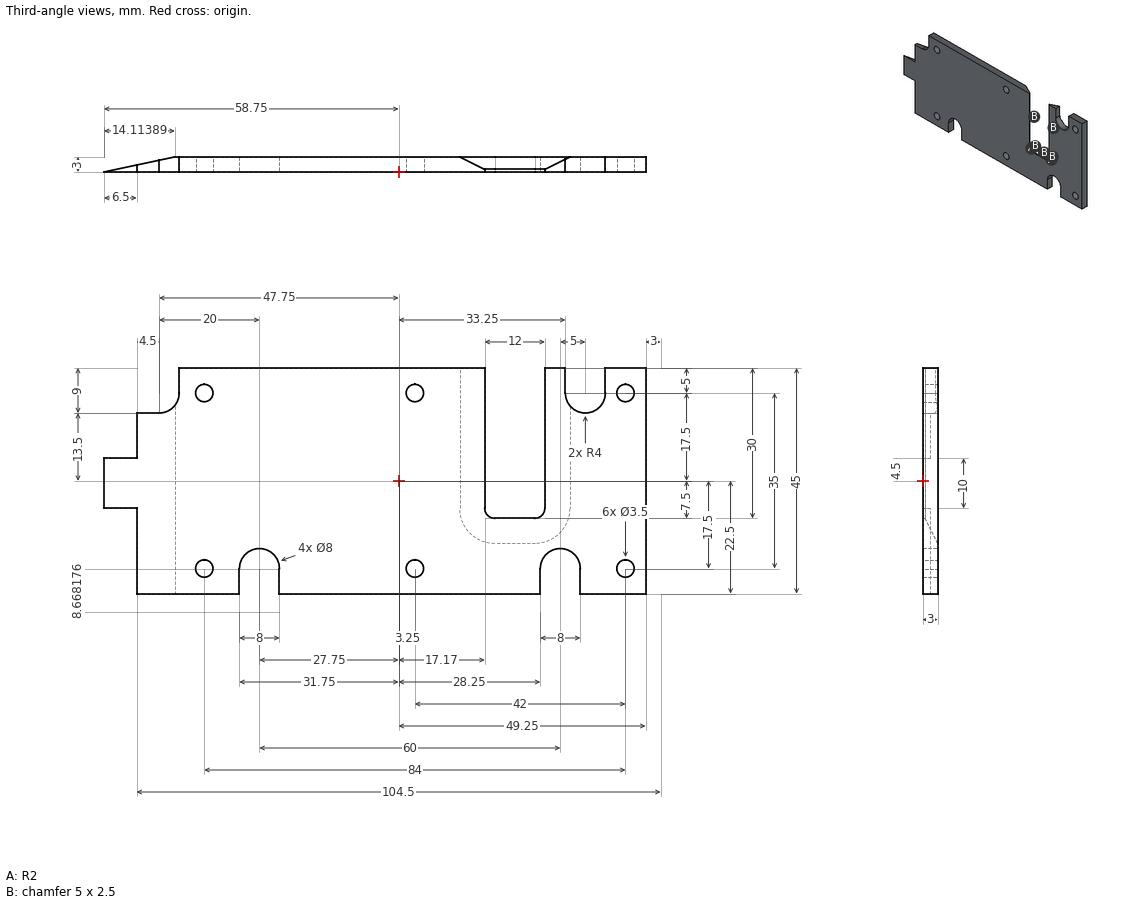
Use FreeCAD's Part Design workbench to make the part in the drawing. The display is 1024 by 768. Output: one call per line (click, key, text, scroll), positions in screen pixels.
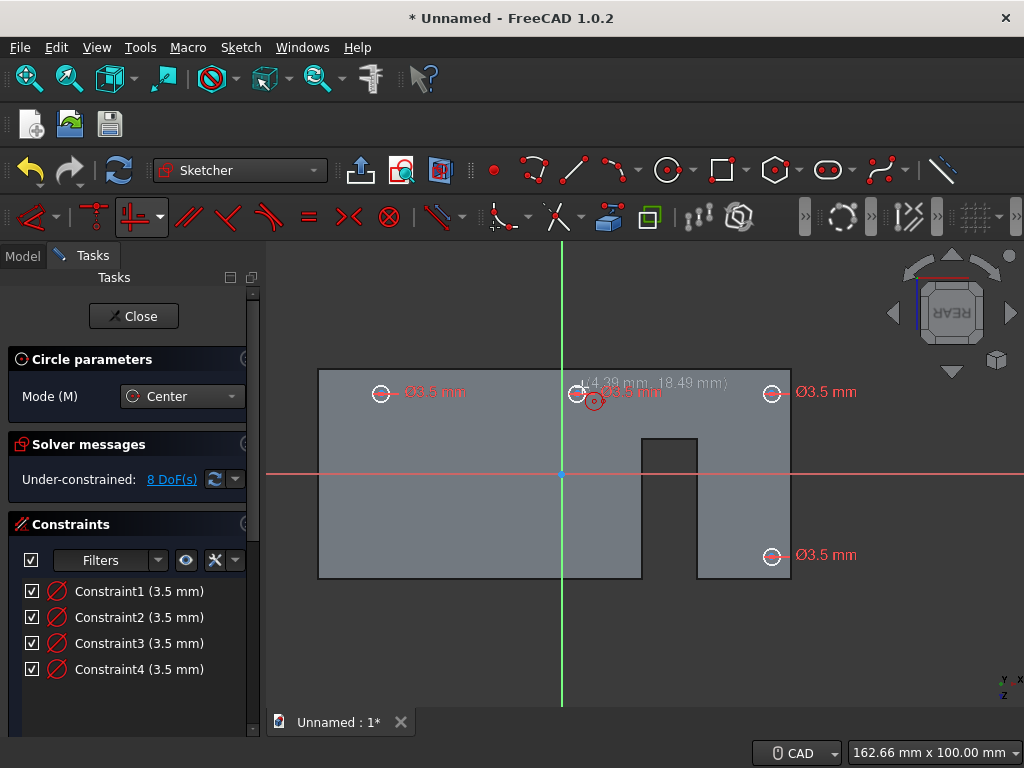
scroll(381, 556, up, 6)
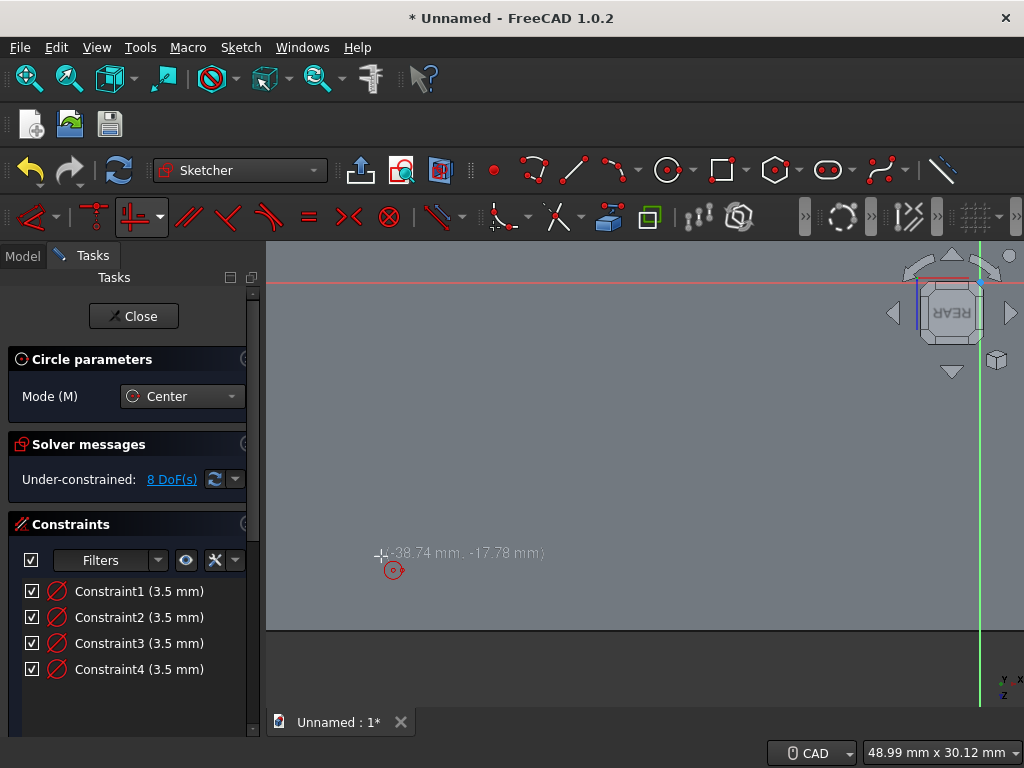
scroll(381, 556, down, 6)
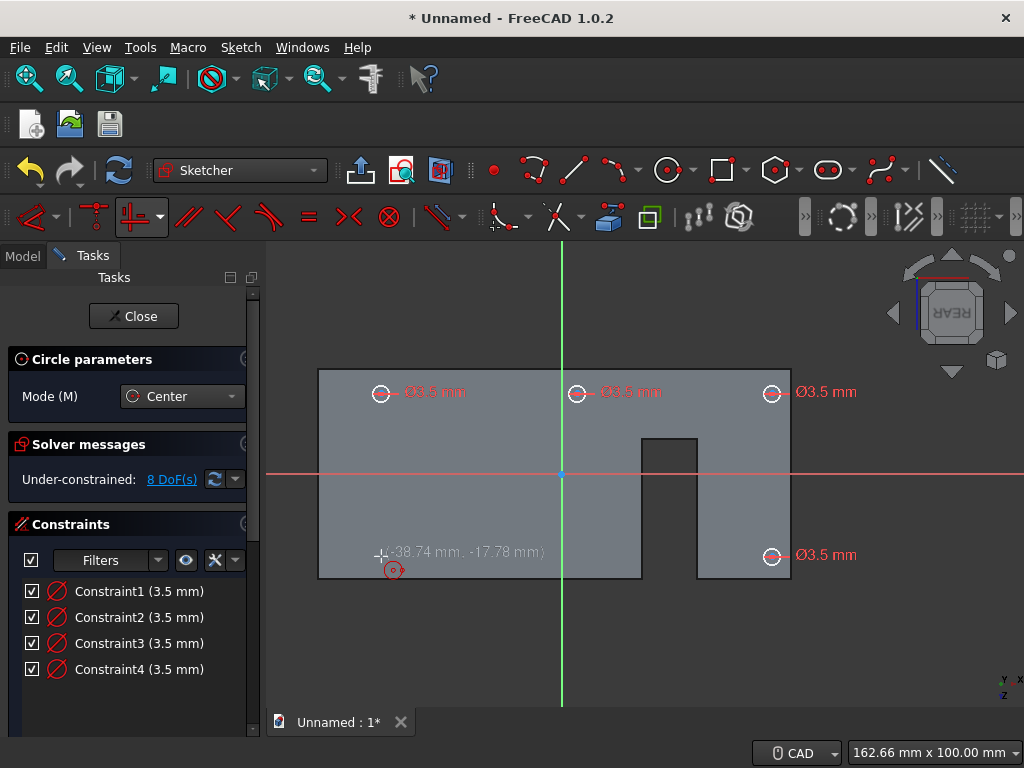
click(381, 556)
move(387, 550)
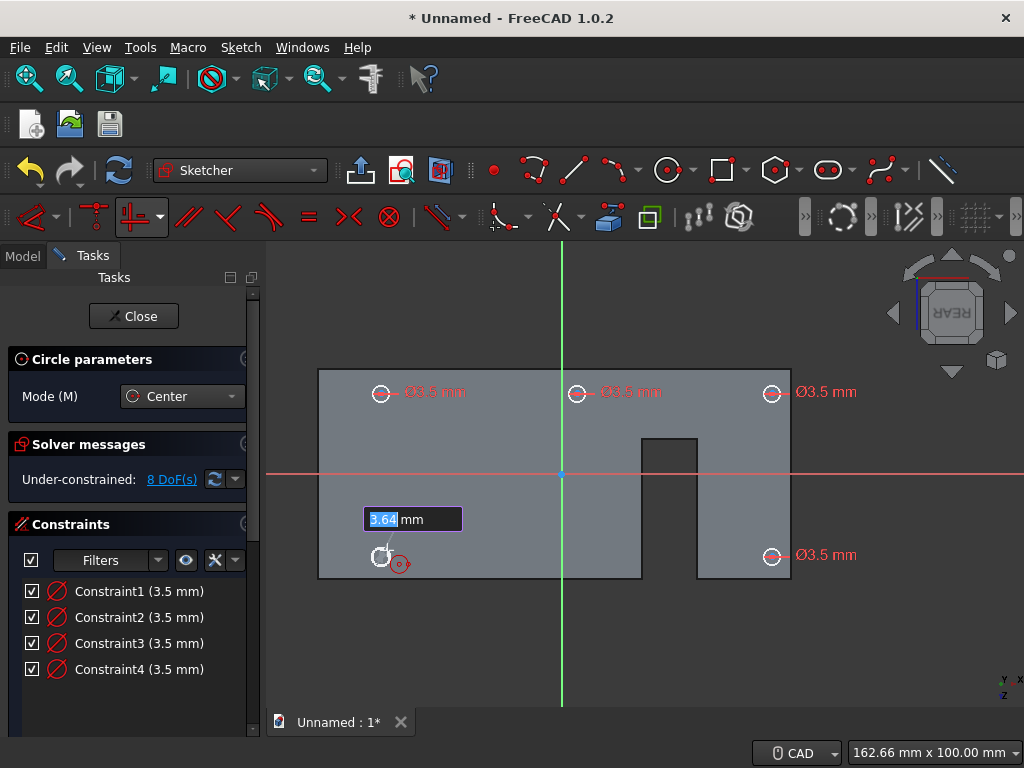
text(3.5)
key(Return)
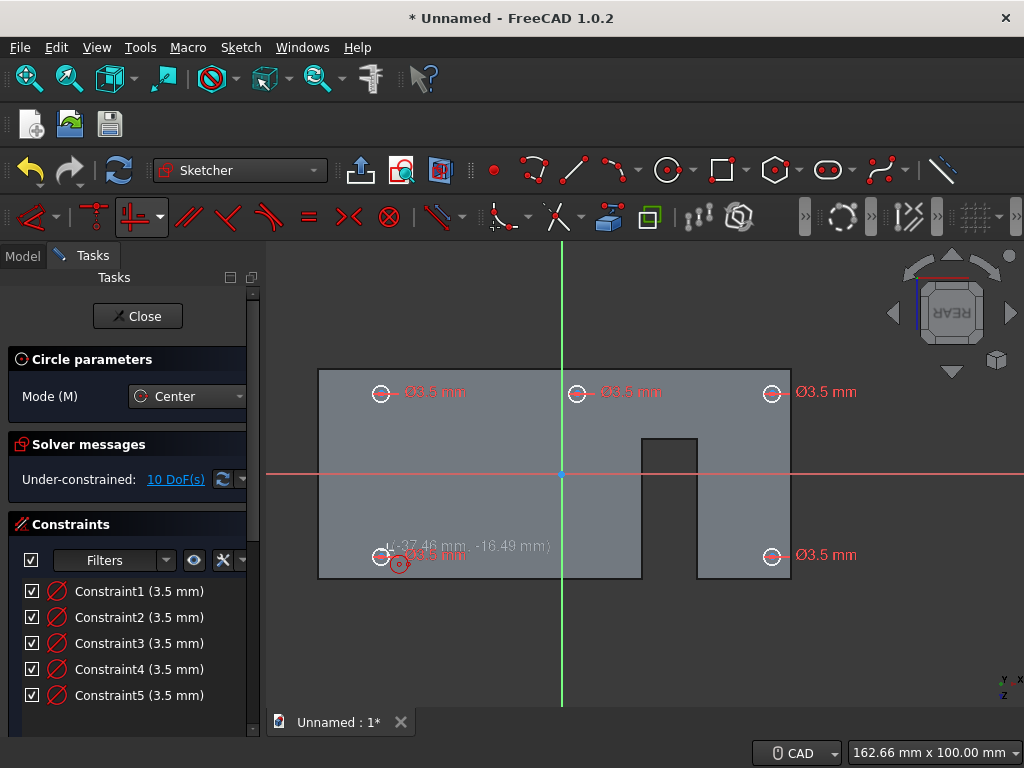
scroll(577, 556, up, 6)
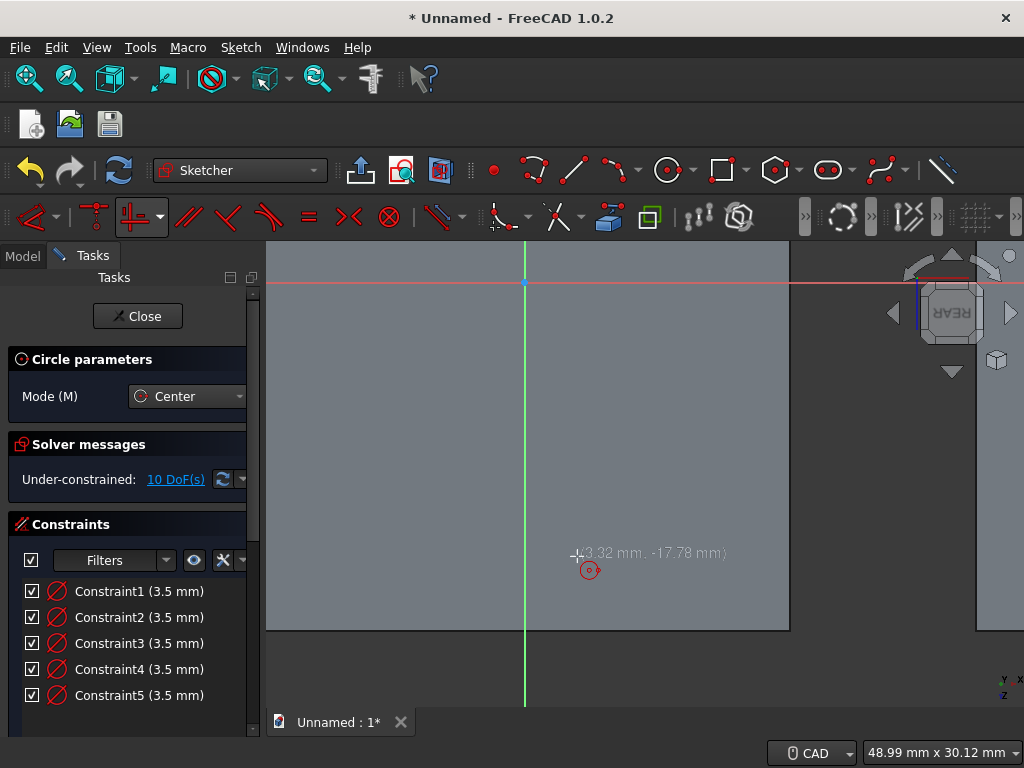
scroll(577, 556, down, 6)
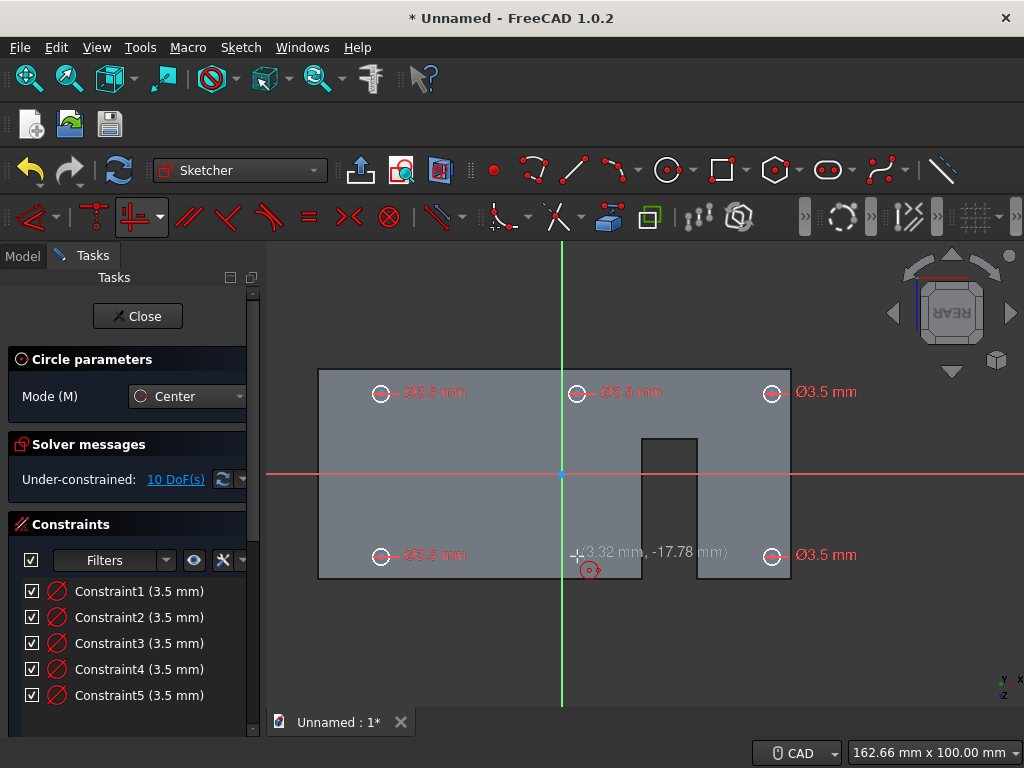
click(577, 556)
move(582, 550)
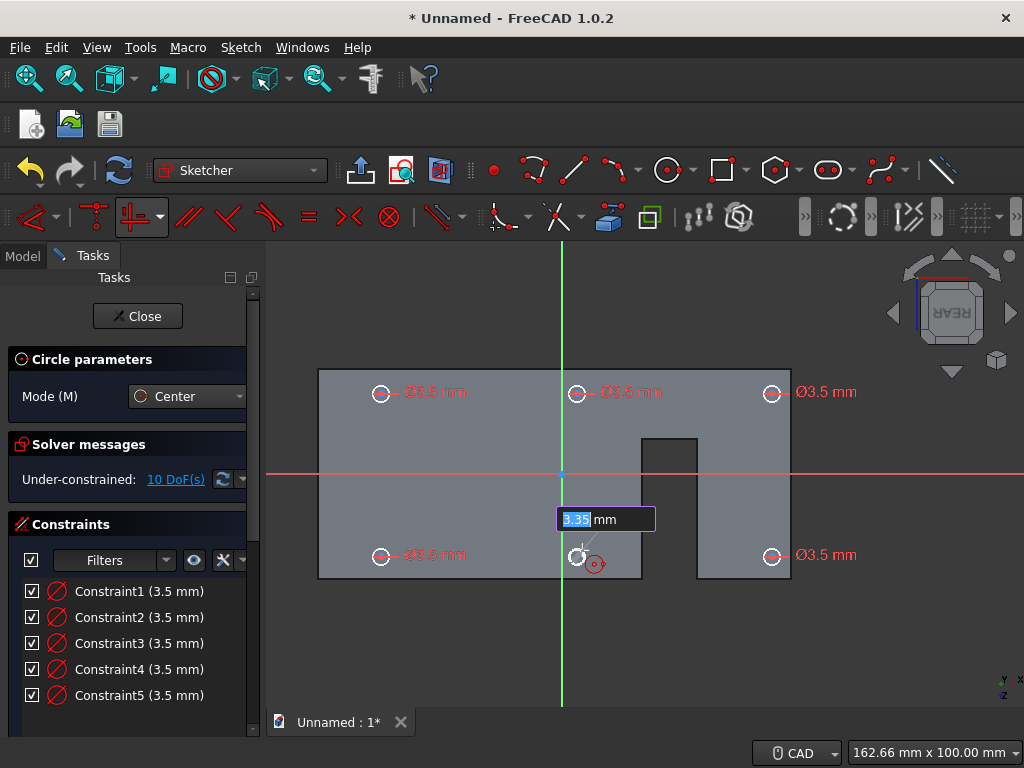
text(3.5)
key(Return)
key(Escape)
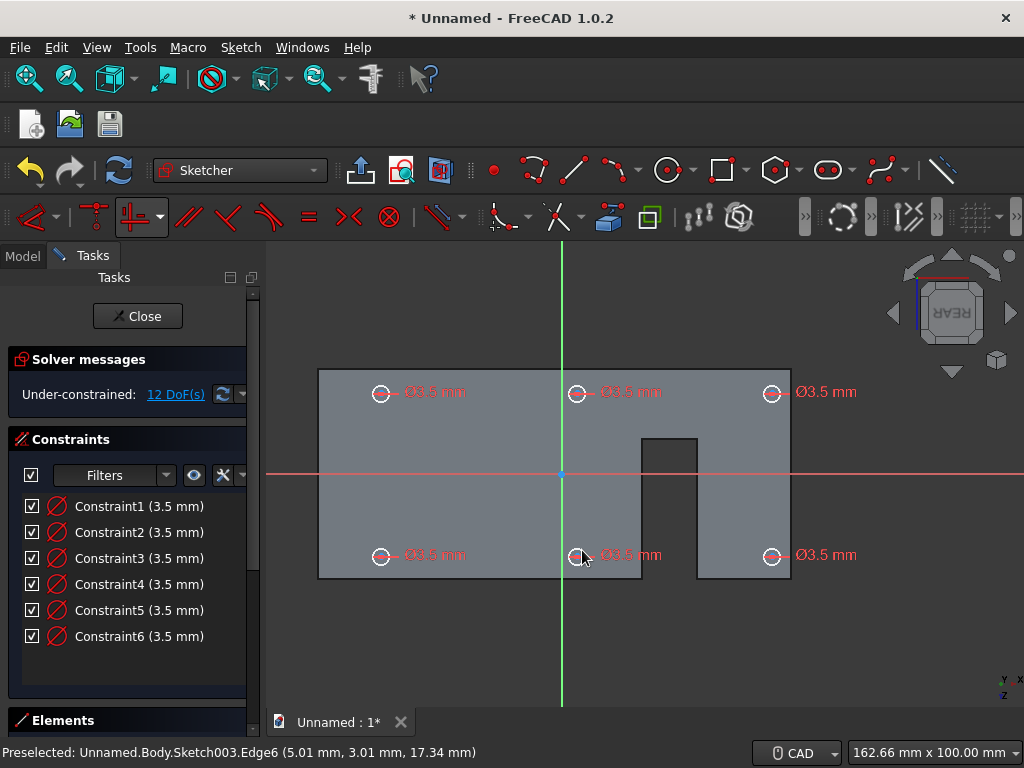
click(772, 394)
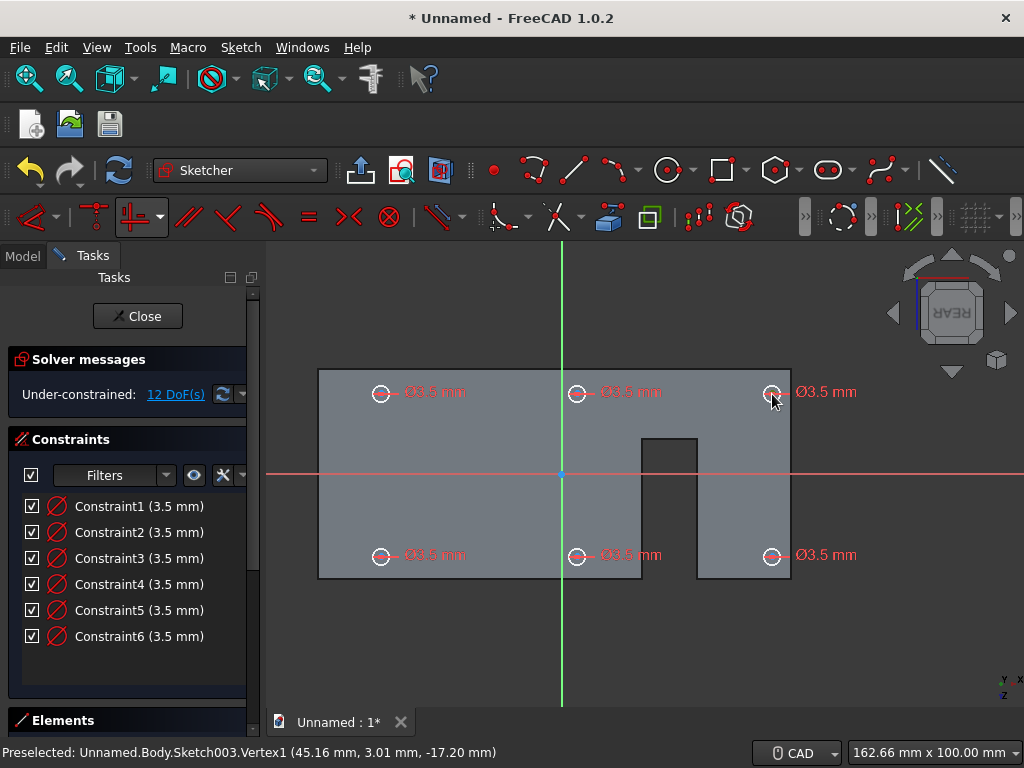
click(772, 557)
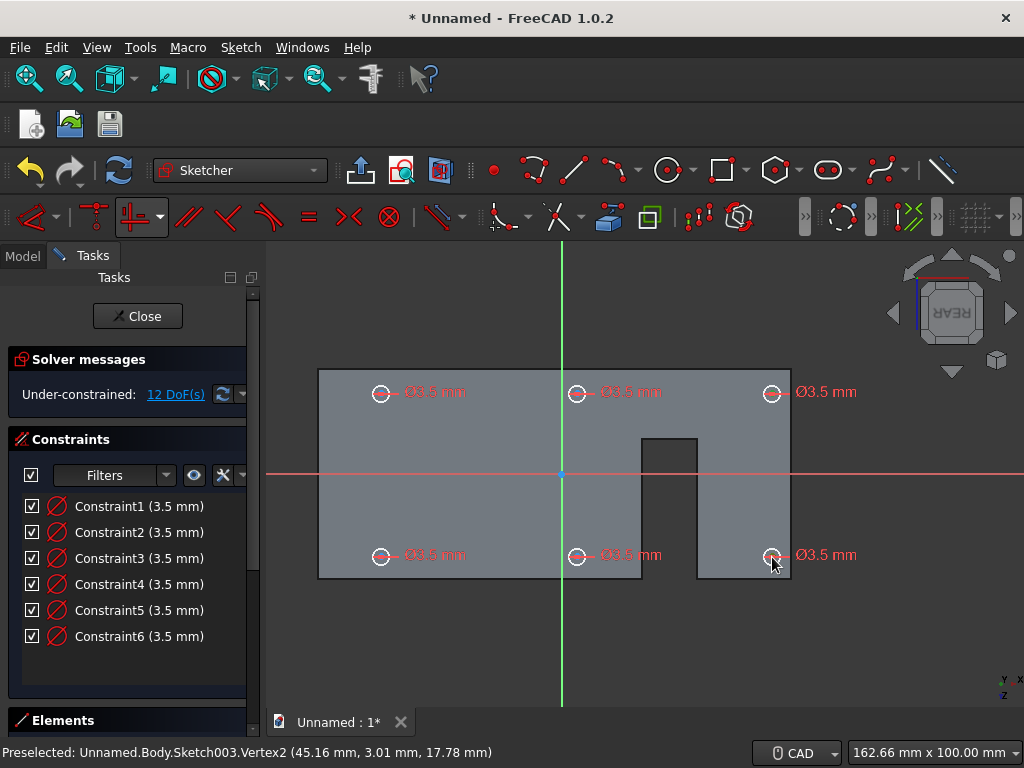
key(v)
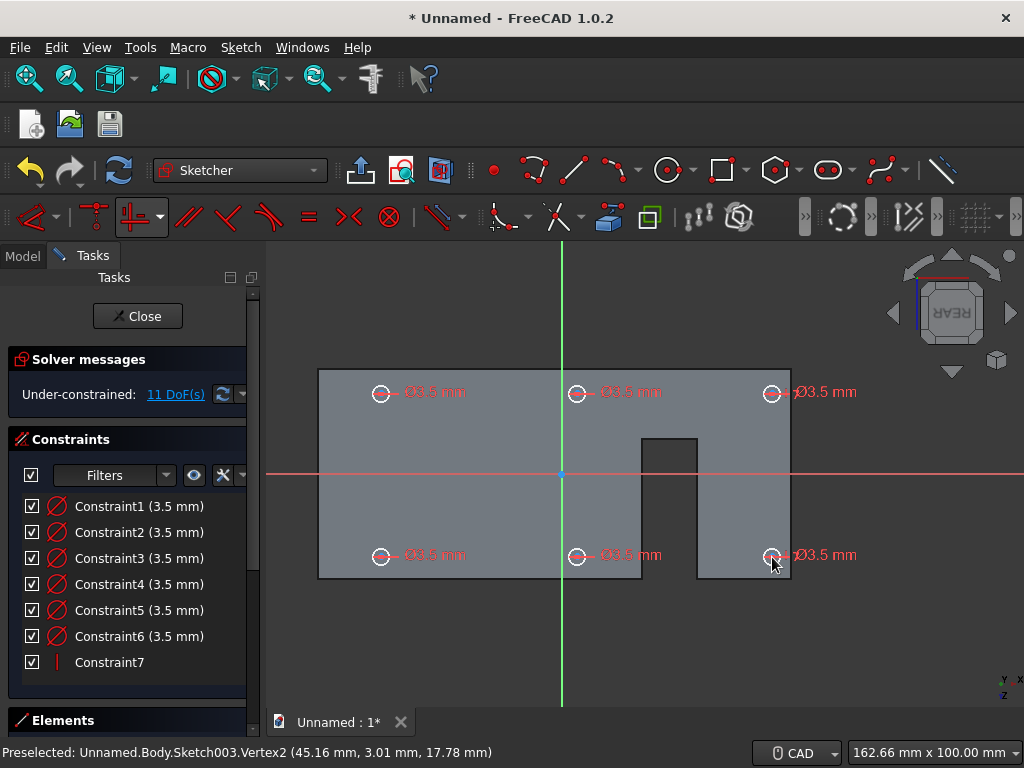
click(772, 394)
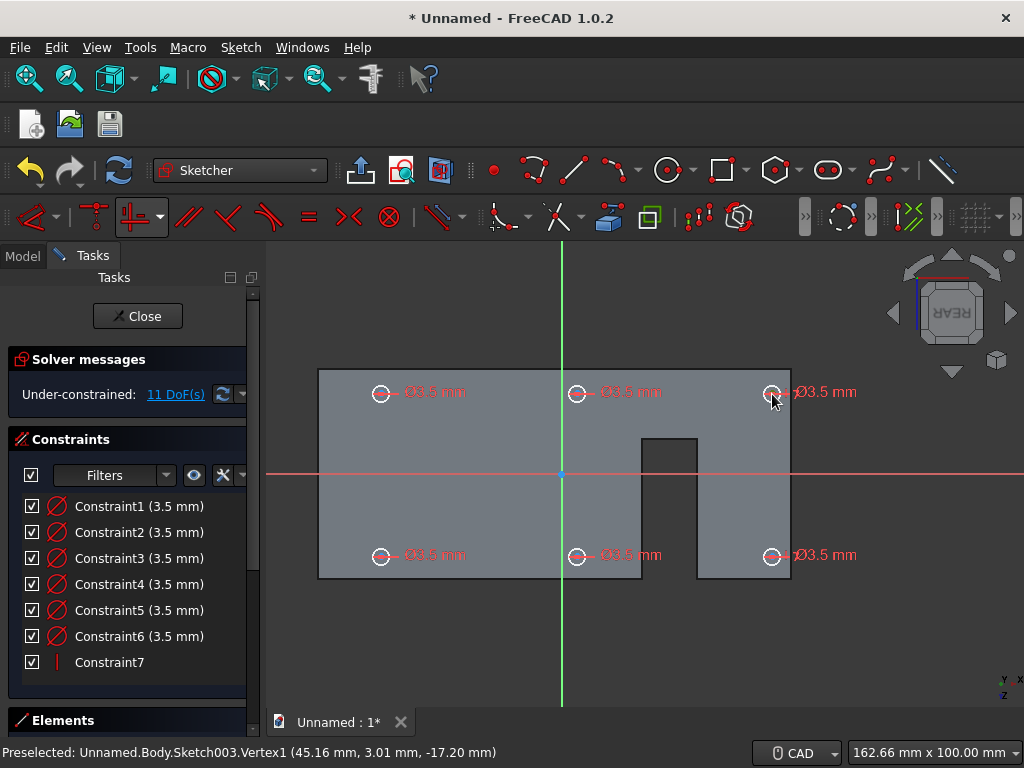
click(381, 394)